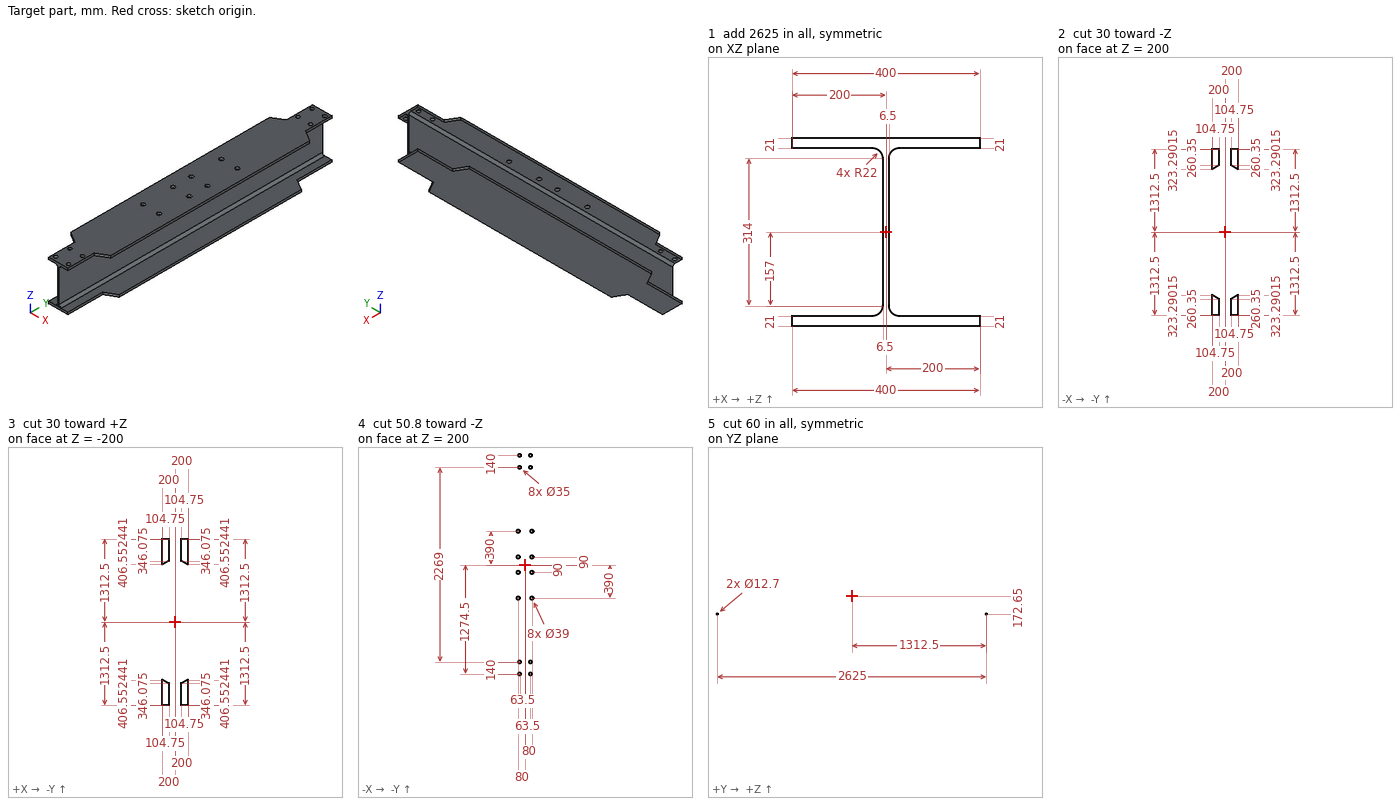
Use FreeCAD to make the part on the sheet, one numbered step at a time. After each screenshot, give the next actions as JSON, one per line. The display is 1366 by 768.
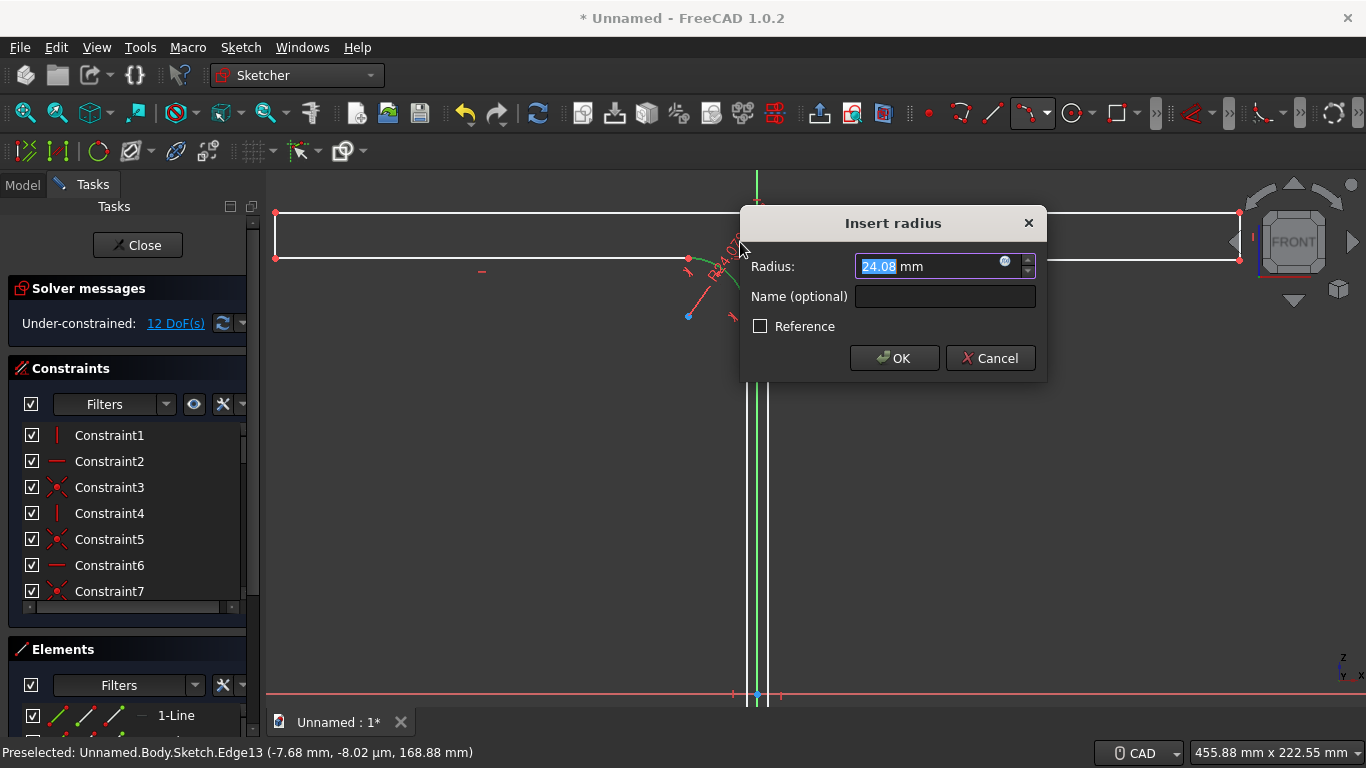
{"action": "type", "text": "22"}
{"action": "key", "text": "Return"}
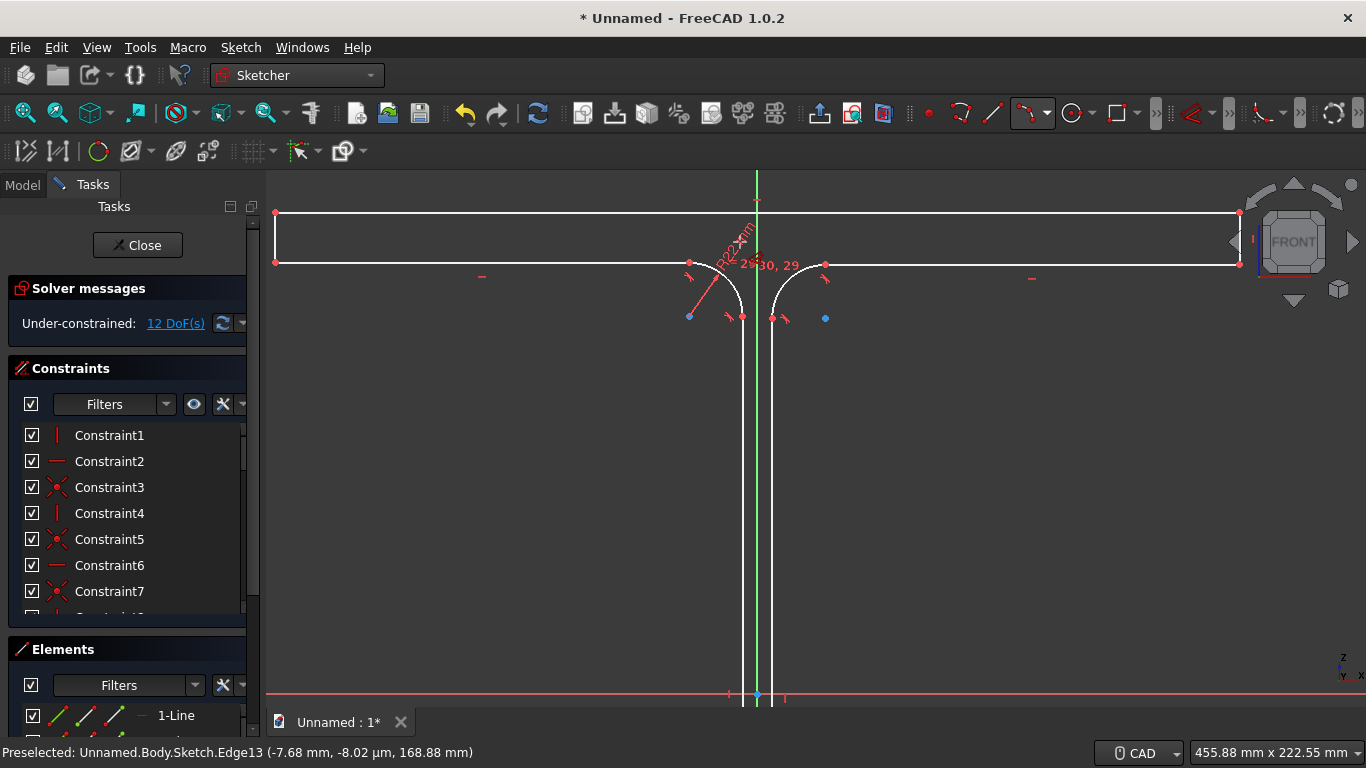
{"action": "scroll", "coordinate": [742, 290], "scroll_direction": "down", "scroll_amount": 5}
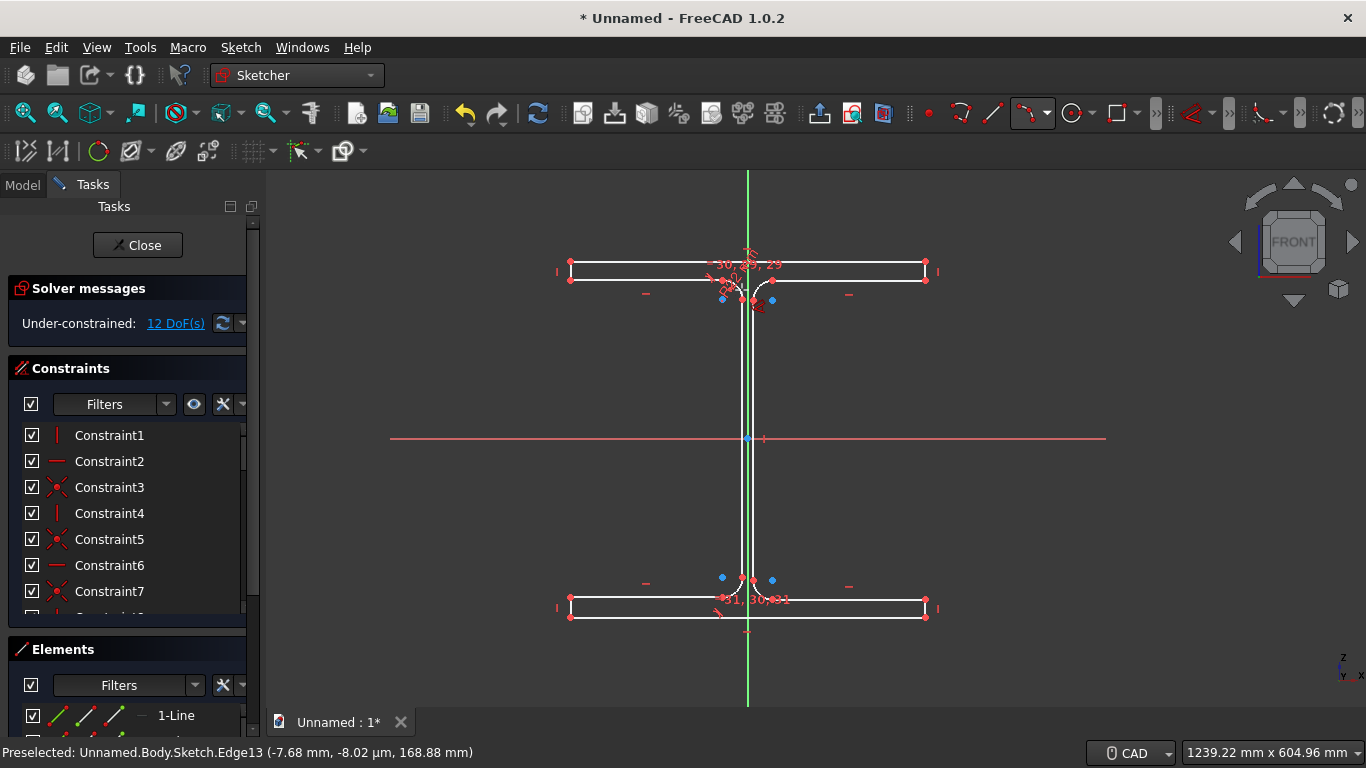
{"action": "scroll", "coordinate": [571, 275], "scroll_direction": "up", "scroll_amount": 5}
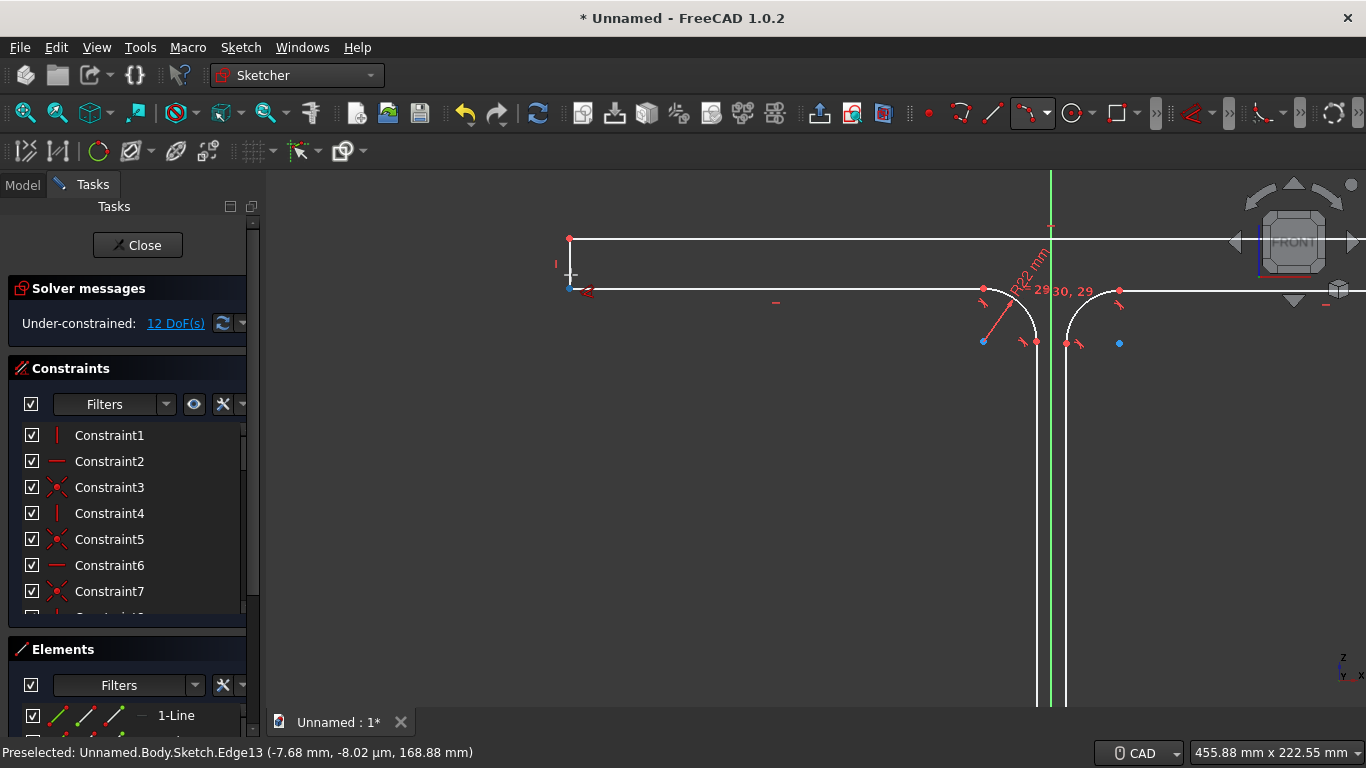
{"action": "left_click", "coordinate": [570, 274]}
{"action": "left_click", "coordinate": [536, 264]}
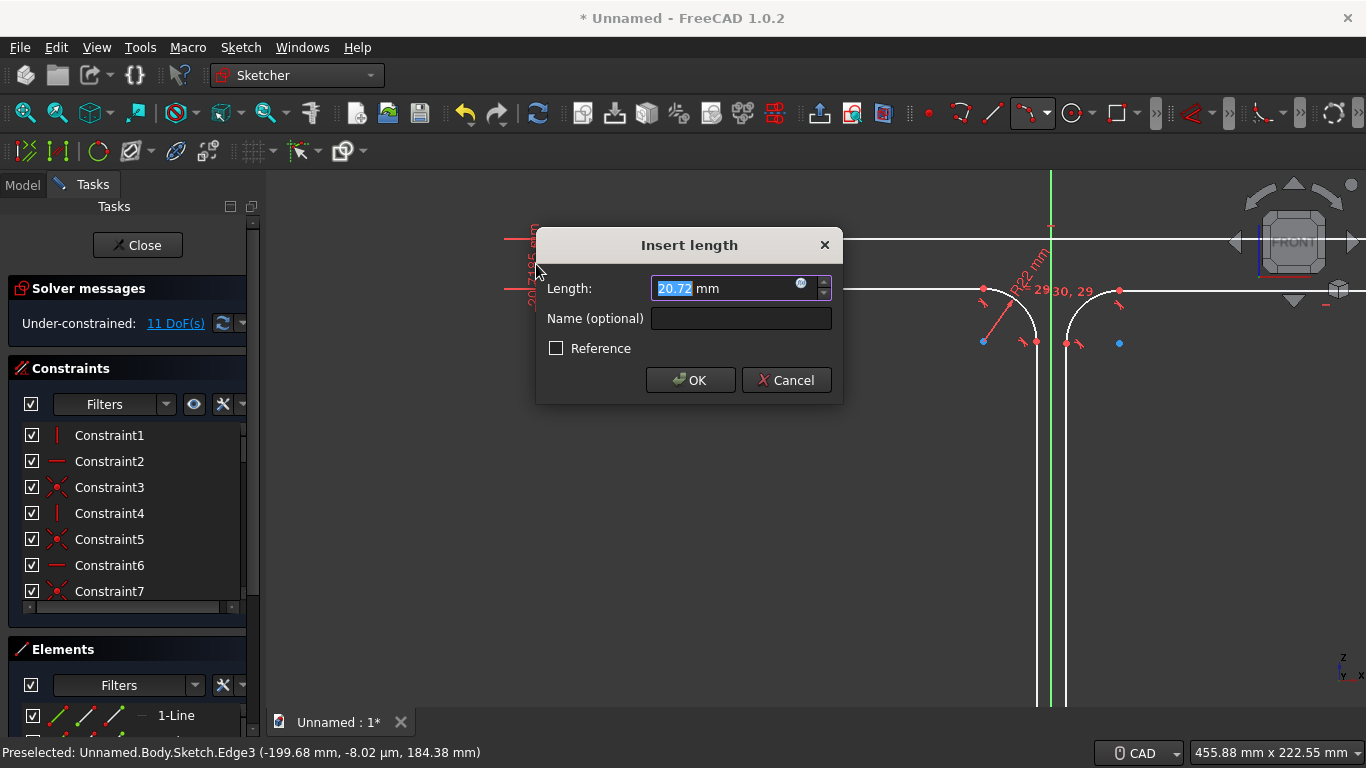
{"action": "type", "text": "21"}
{"action": "key", "text": "Return"}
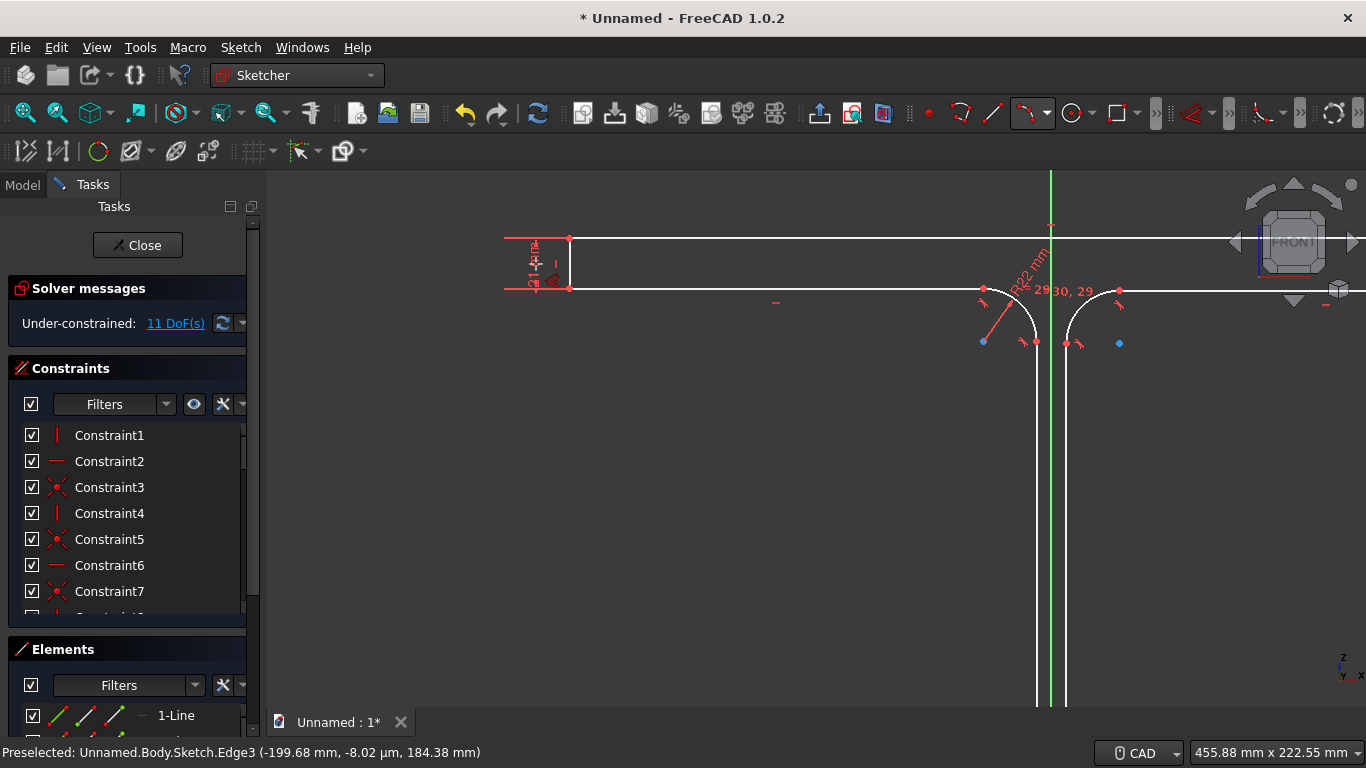
{"action": "scroll", "coordinate": [571, 275], "scroll_direction": "down", "scroll_amount": 5}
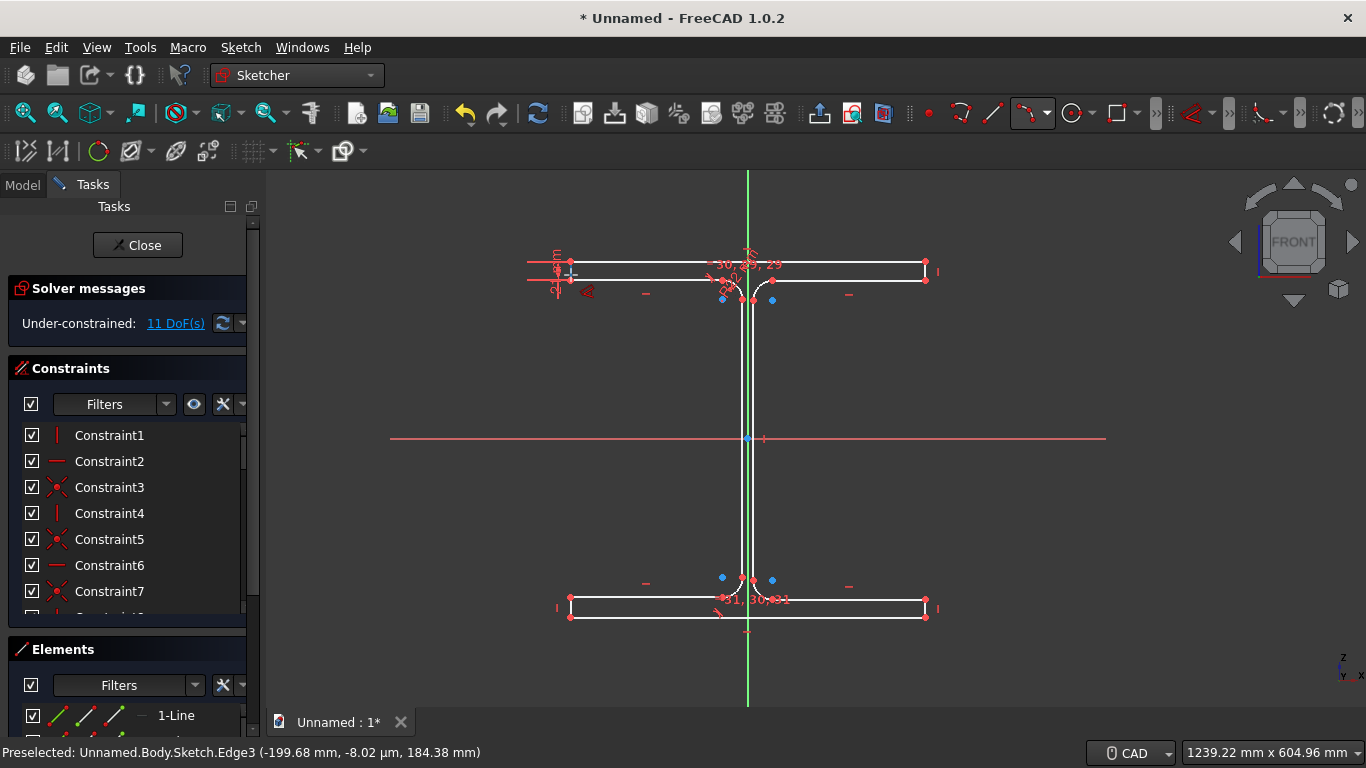
{"action": "scroll", "coordinate": [925, 267], "scroll_direction": "up", "scroll_amount": 5}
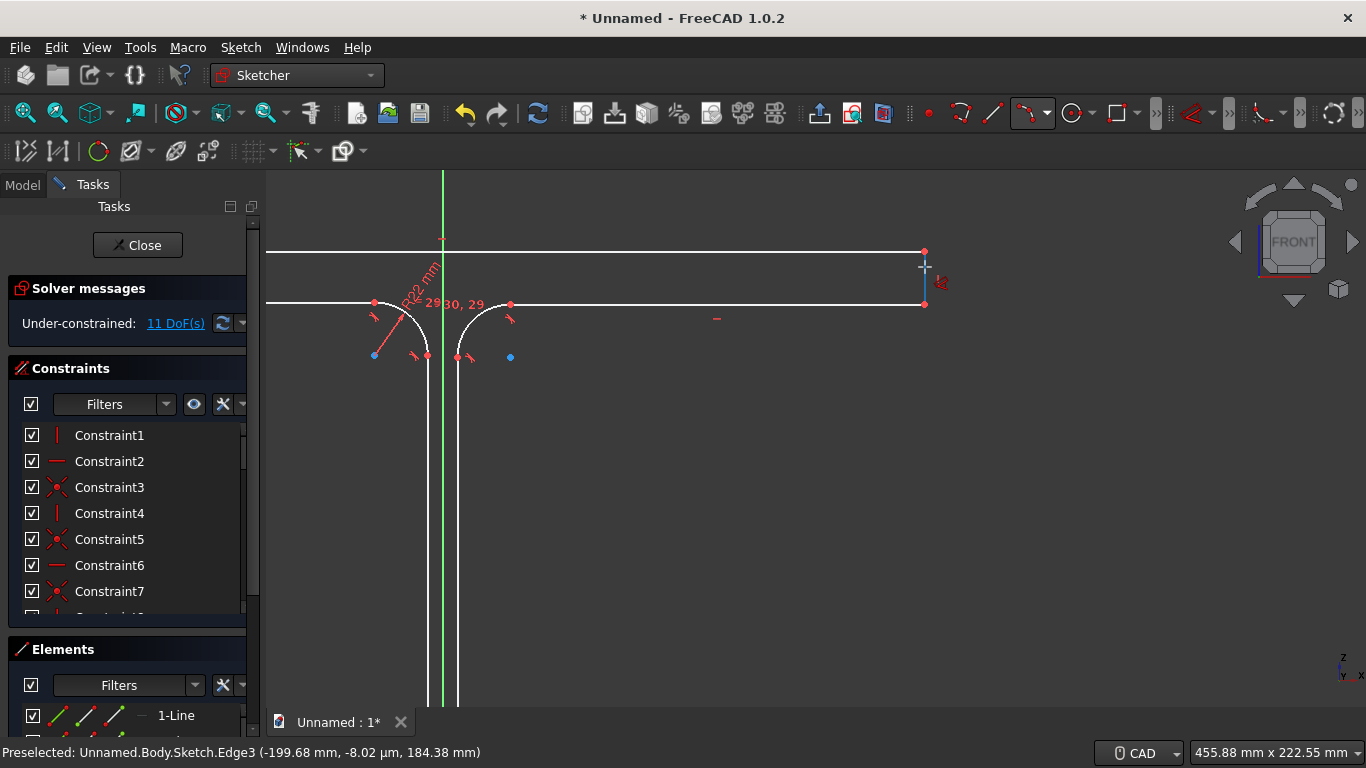
{"action": "left_click", "coordinate": [925, 268]}
{"action": "left_click", "coordinate": [959, 278]}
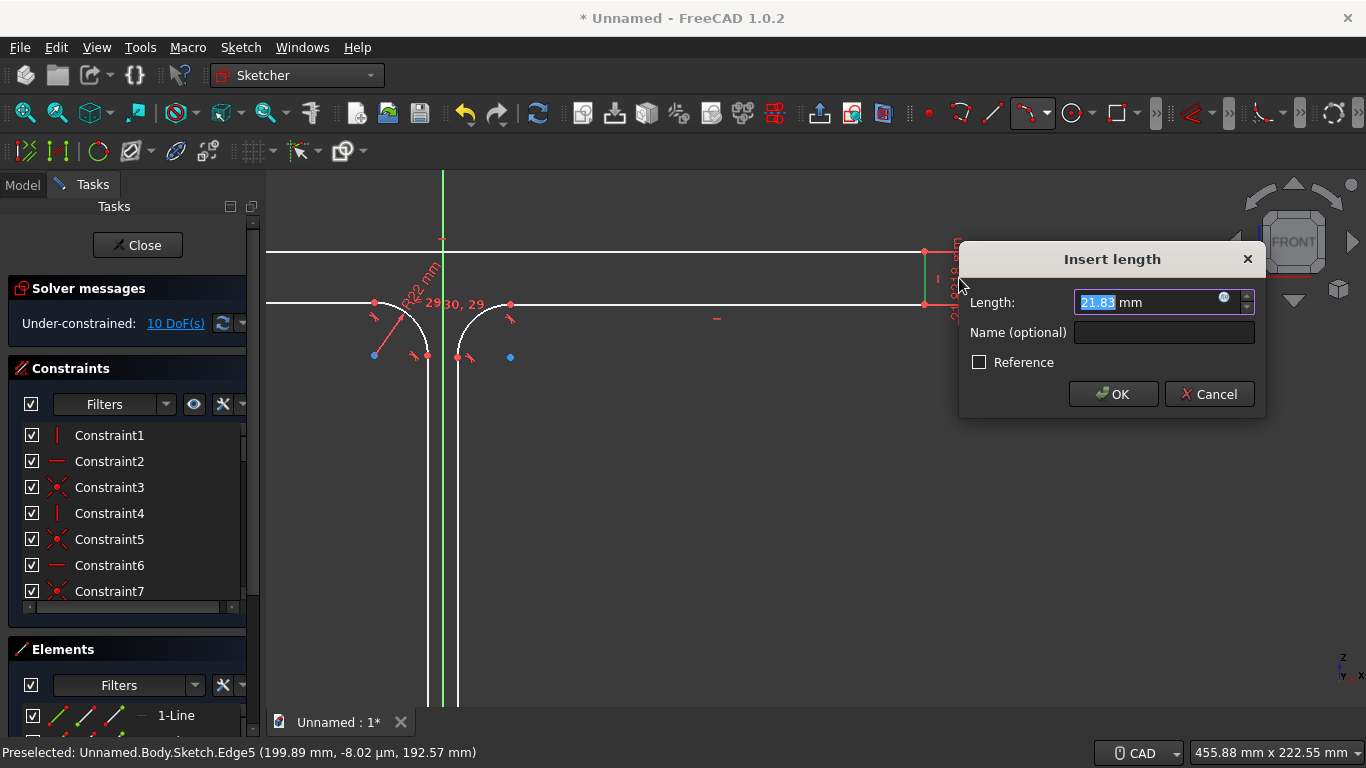
{"action": "type", "text": "21"}
{"action": "key", "text": "Return"}